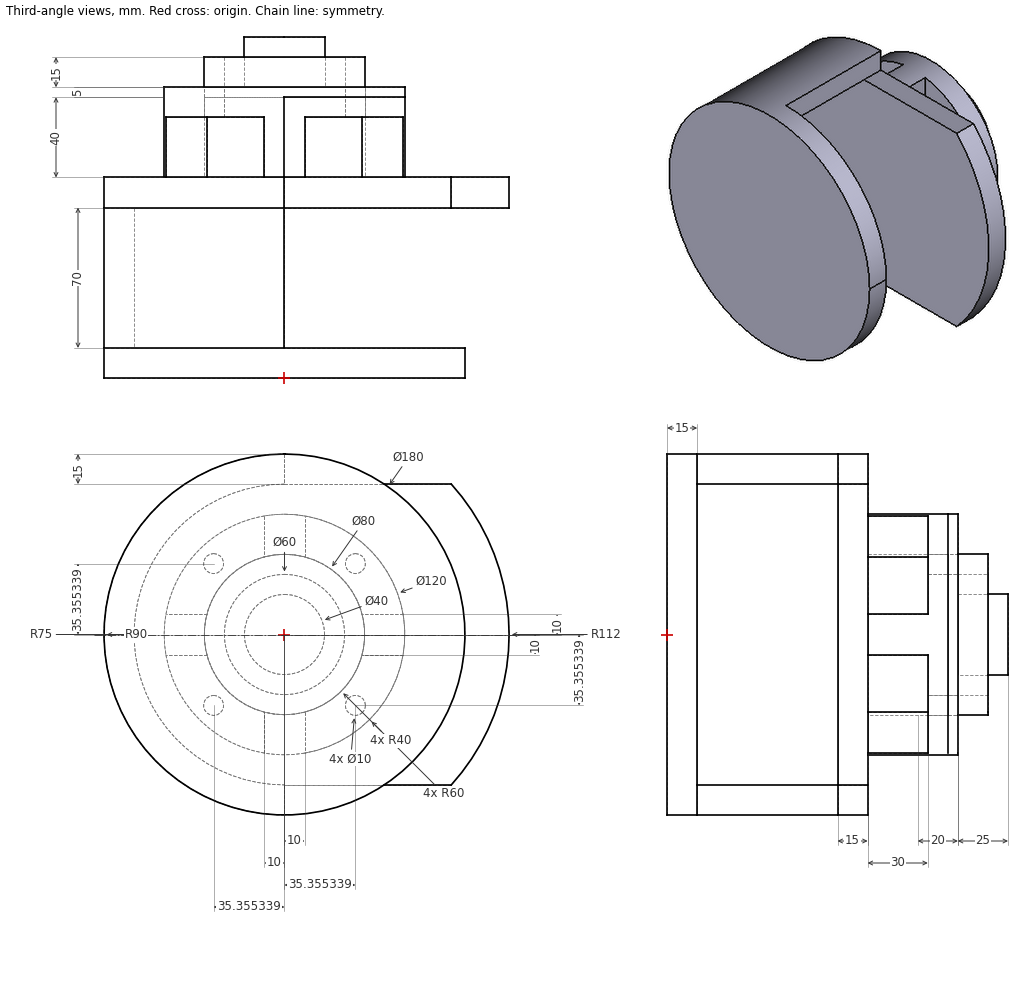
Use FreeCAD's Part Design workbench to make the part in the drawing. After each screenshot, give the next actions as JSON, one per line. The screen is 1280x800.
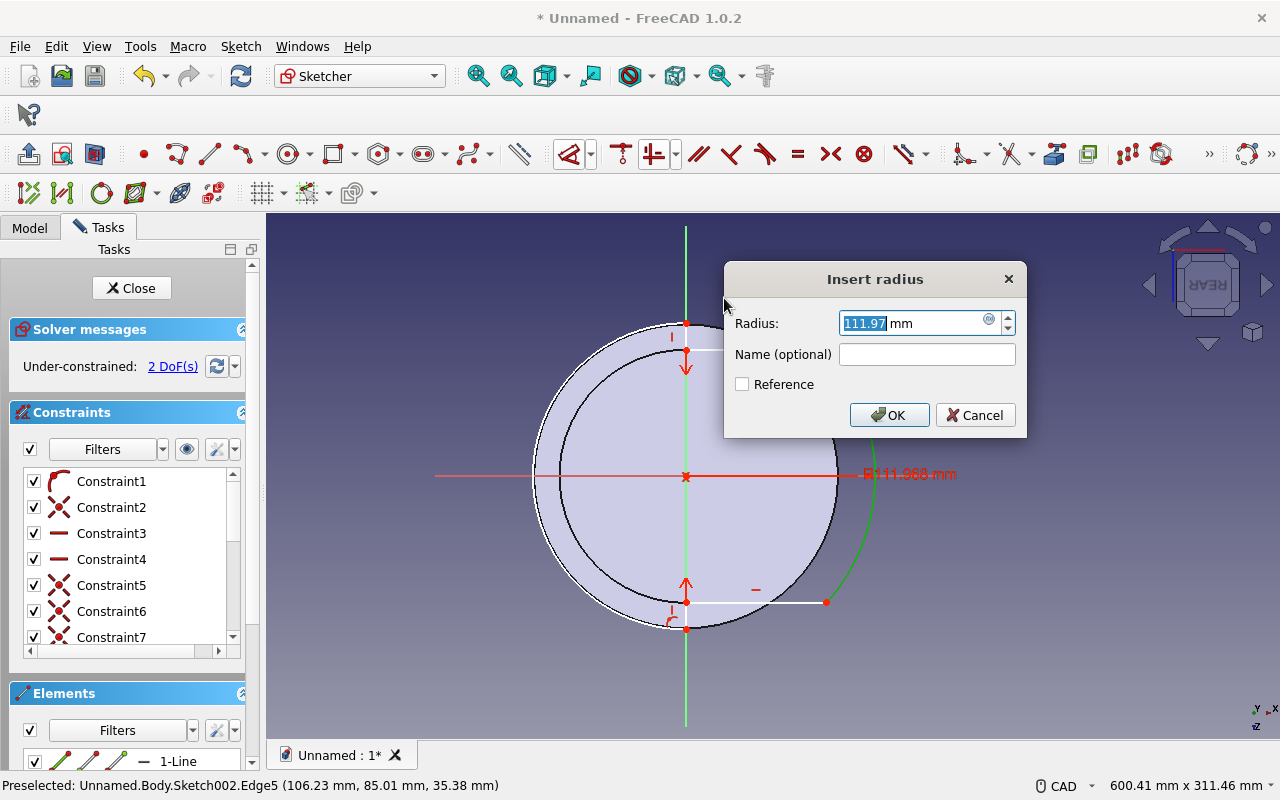
{"action": "type", "text": "112"}
{"action": "key", "text": "Return"}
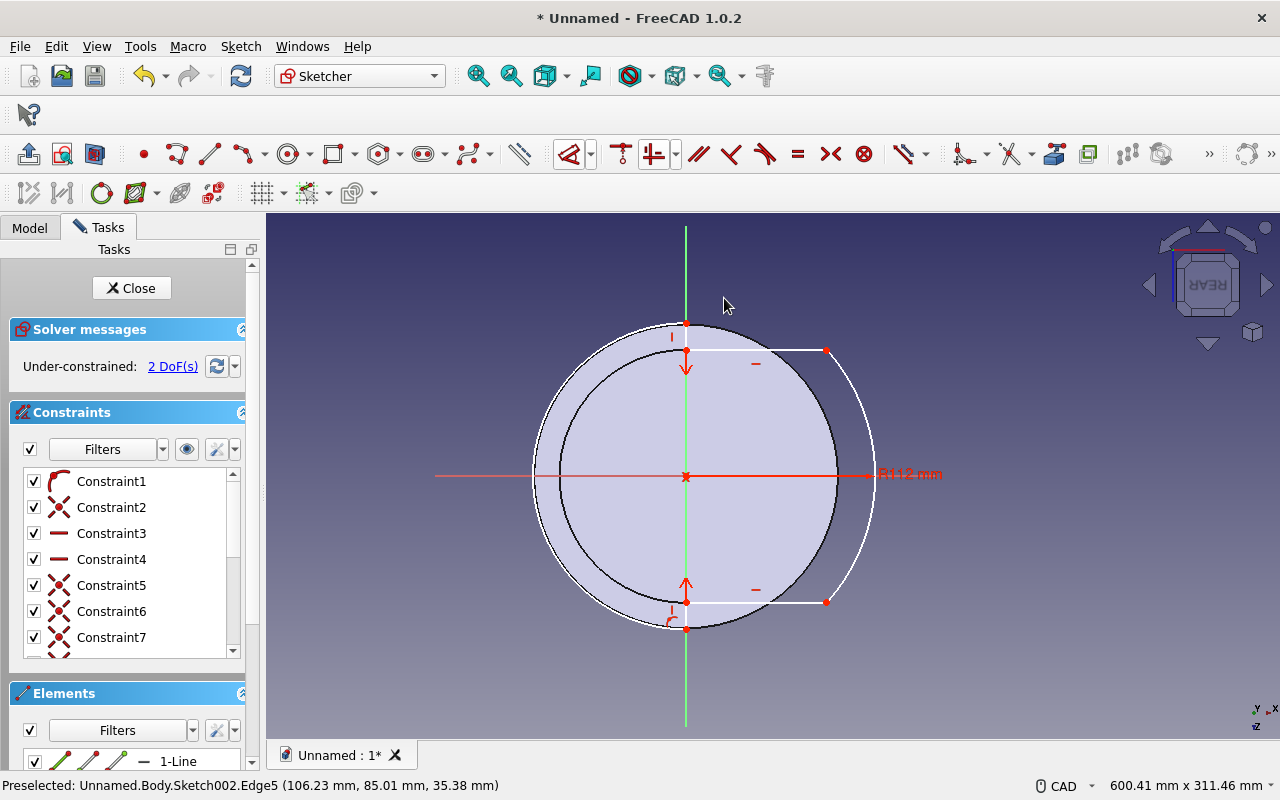
{"action": "left_click", "coordinate": [562, 386]}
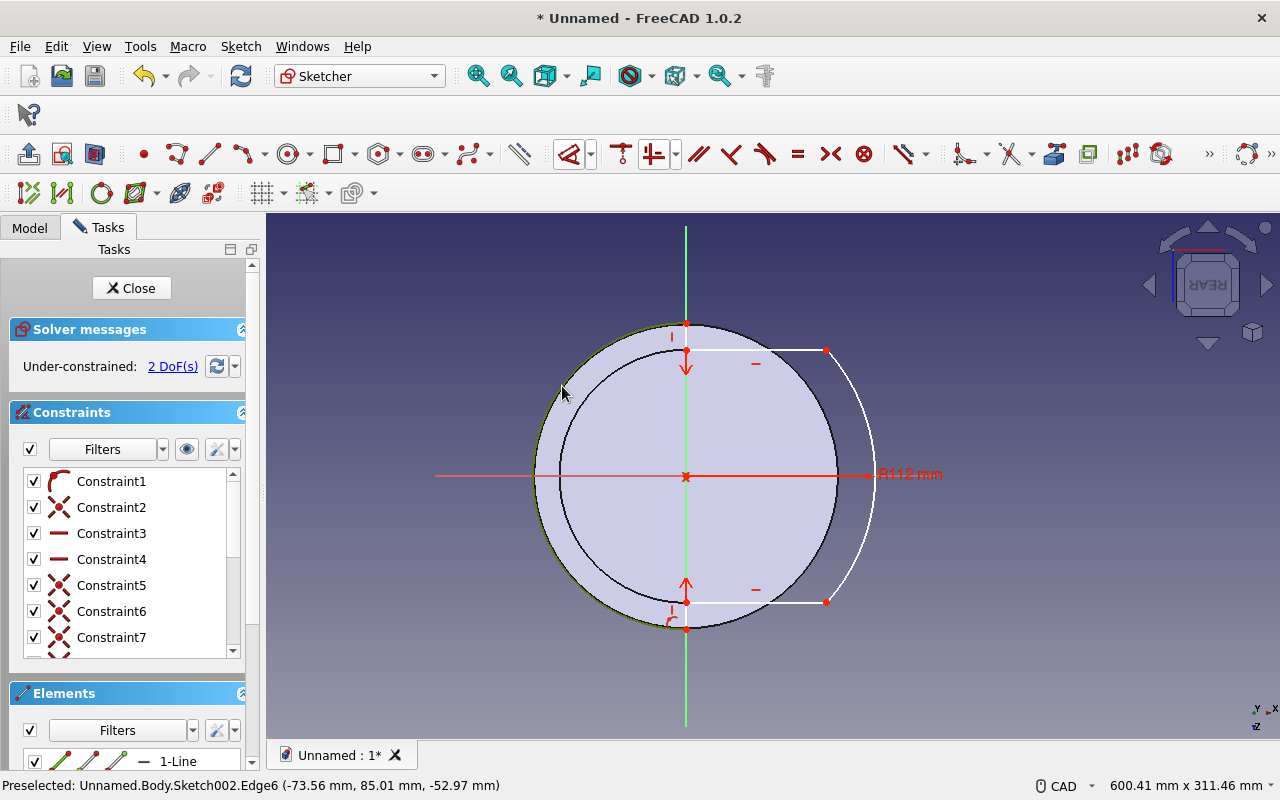
{"action": "key", "text": "k r"}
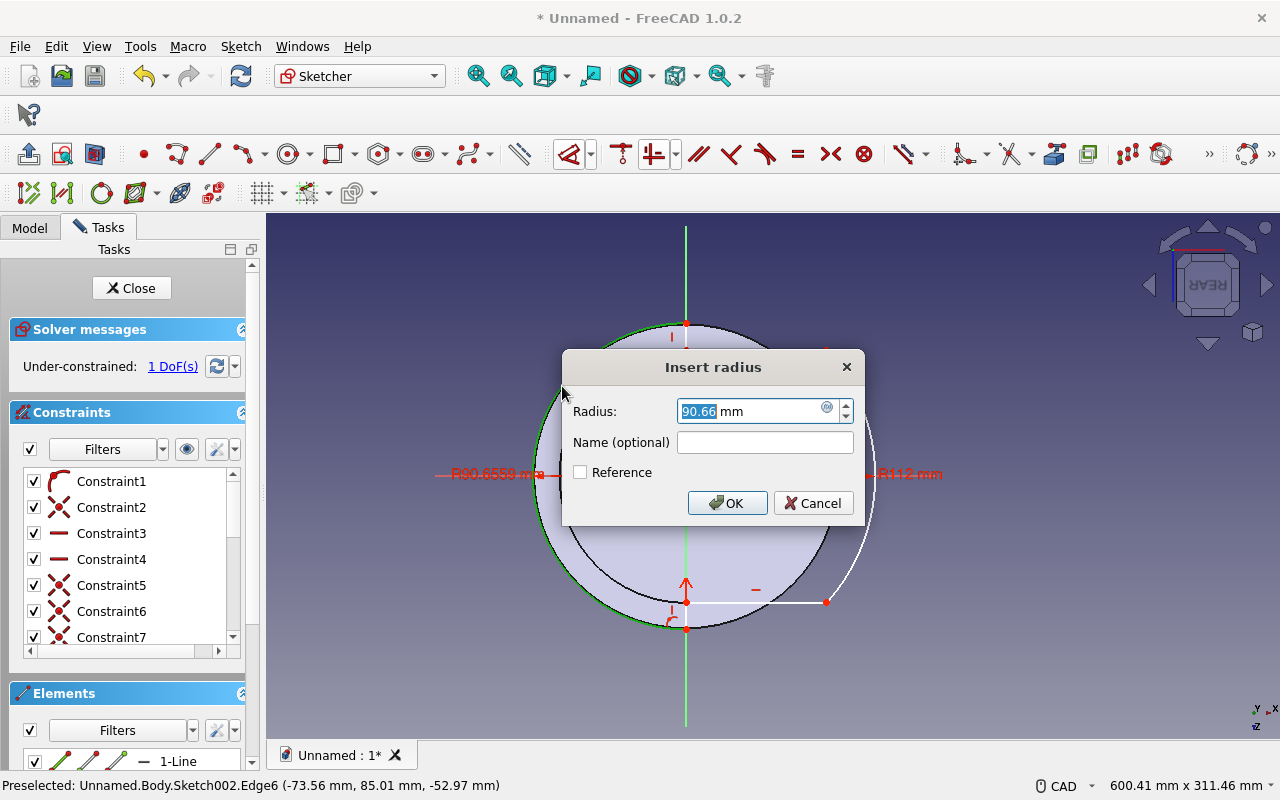
{"action": "type", "text": "90"}
{"action": "key", "text": "Return"}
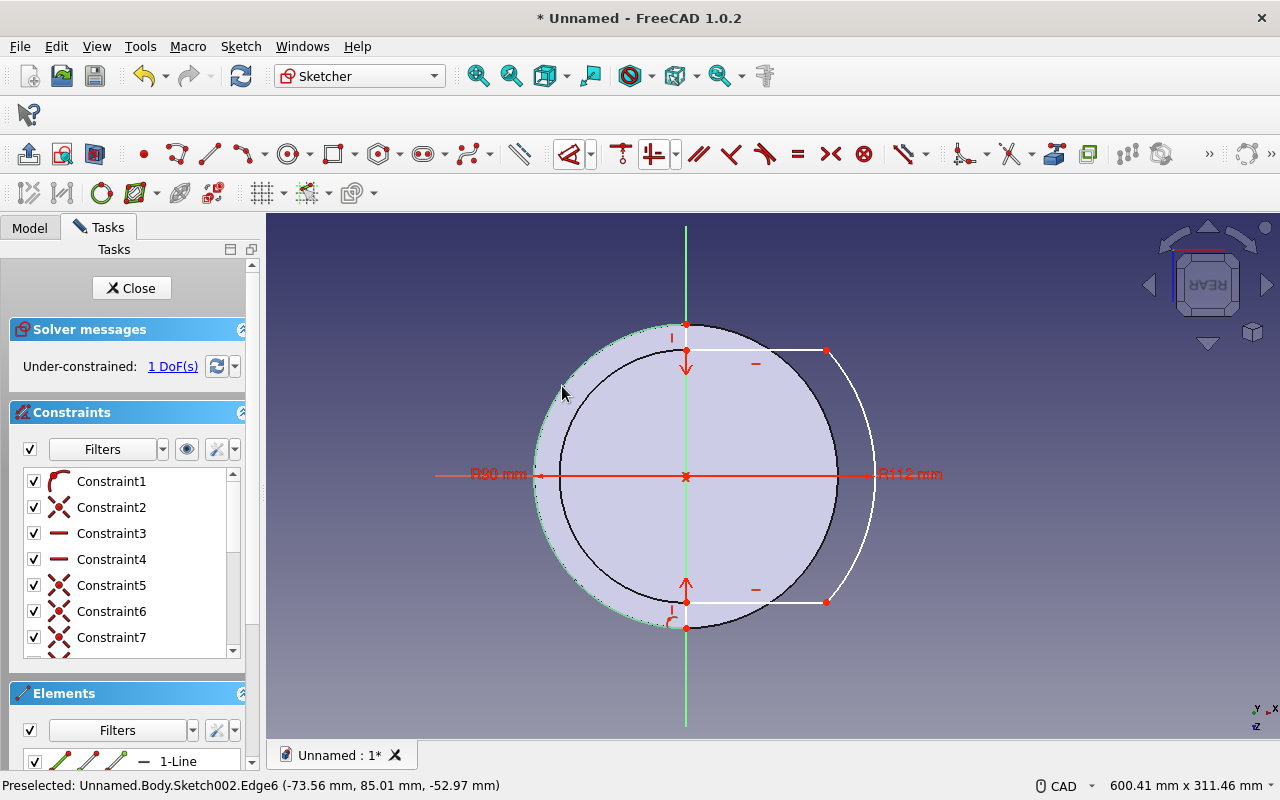
{"action": "scroll", "coordinate": [686, 618], "scroll_direction": "up", "scroll_amount": 3}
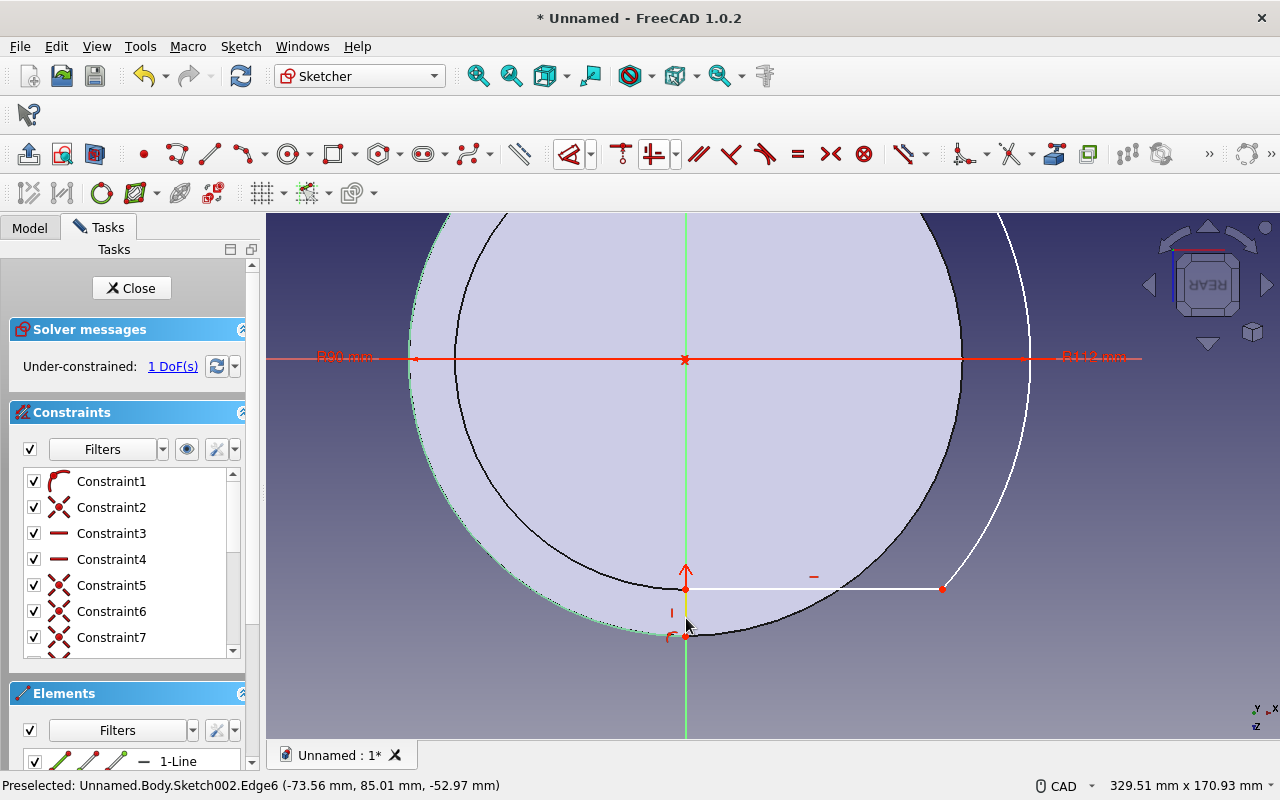
{"action": "left_click", "coordinate": [686, 617]}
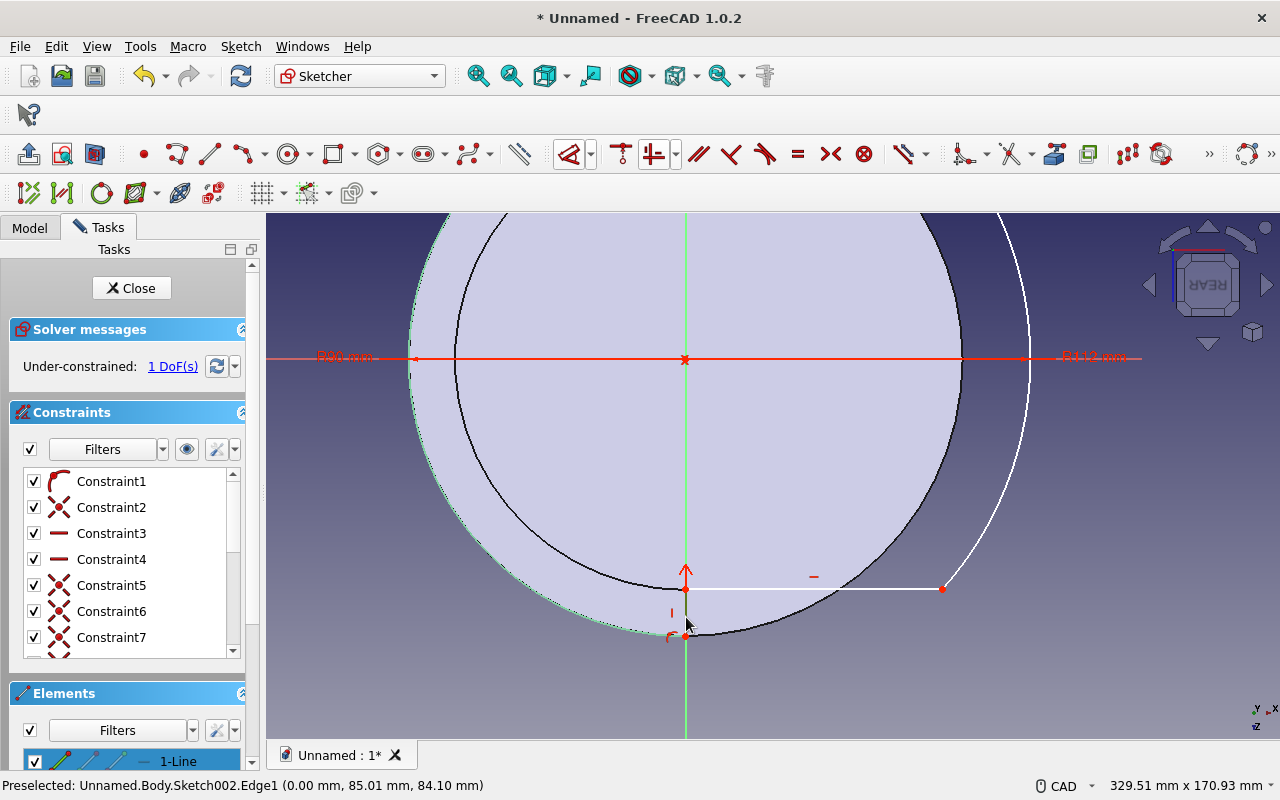
{"action": "key", "text": "i"}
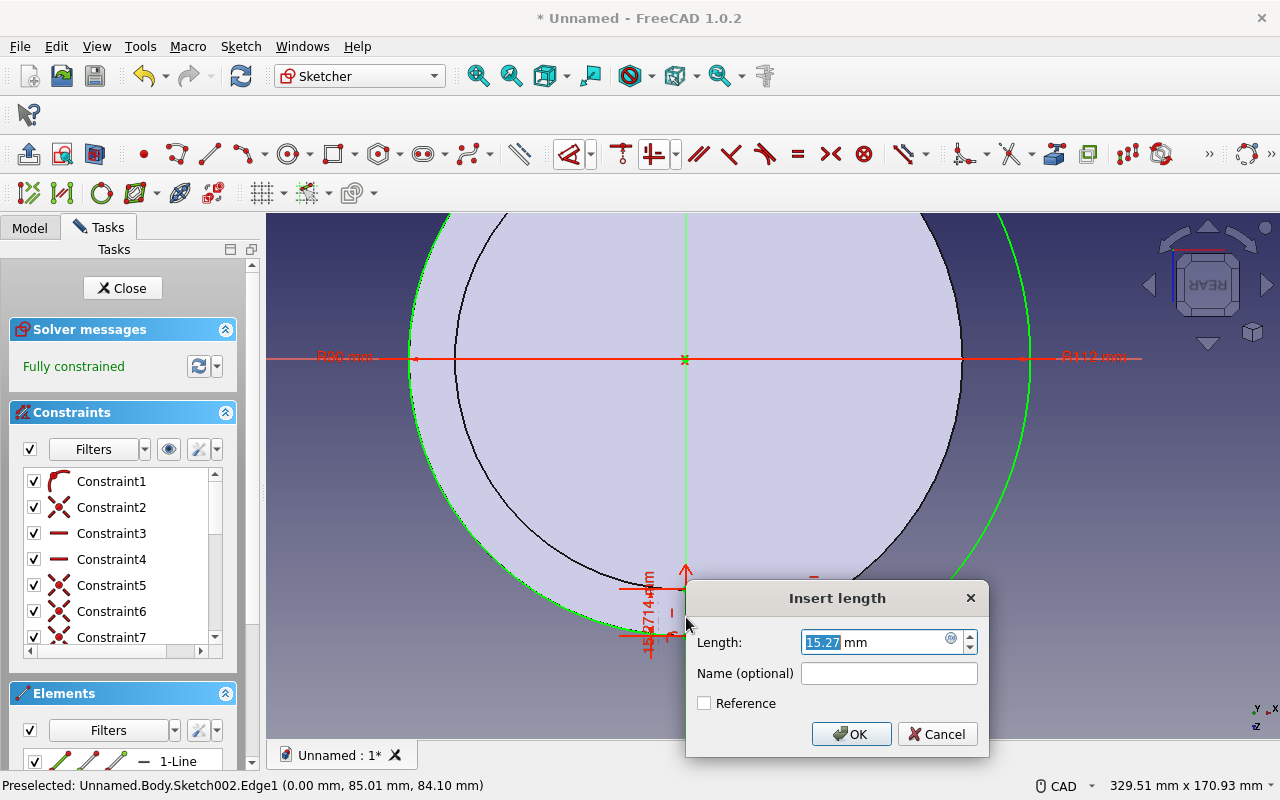
{"action": "type", "text": "15"}
{"action": "key", "text": "Return"}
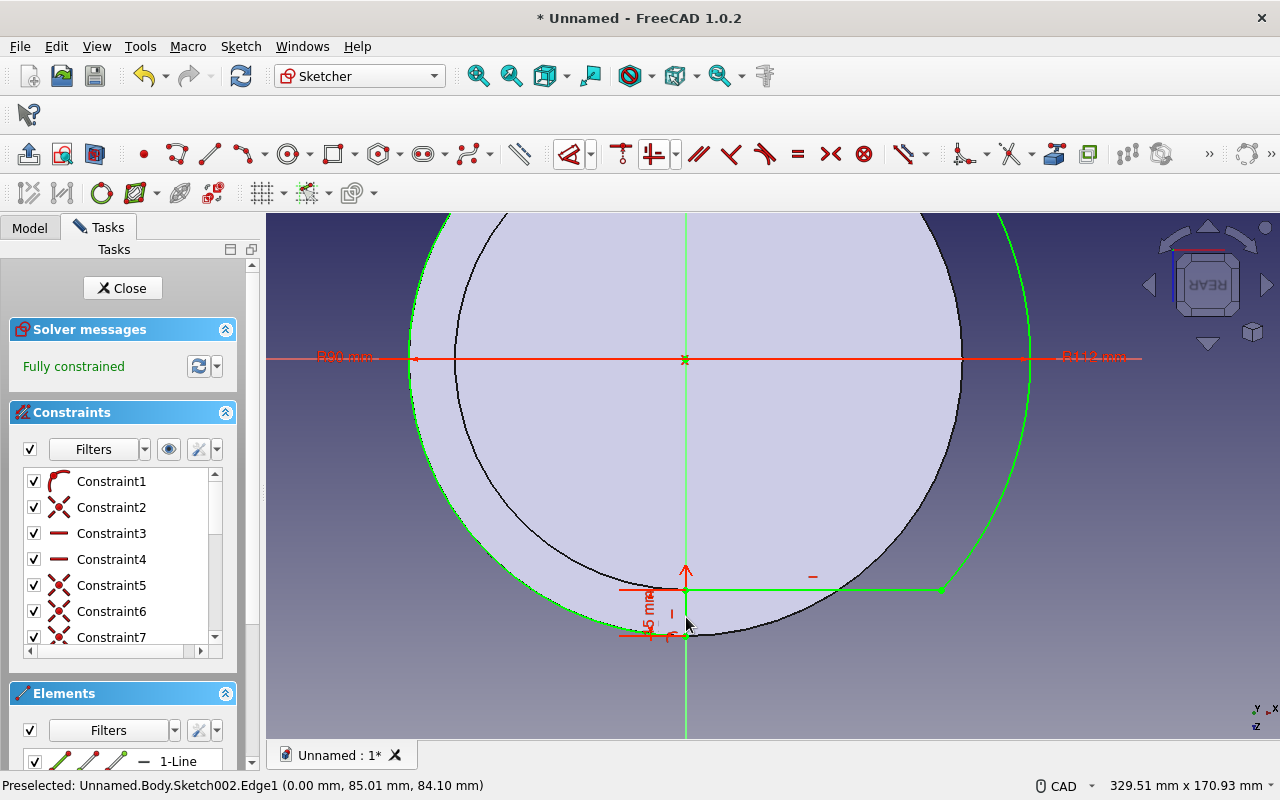
{"action": "left_click", "coordinate": [123, 288]}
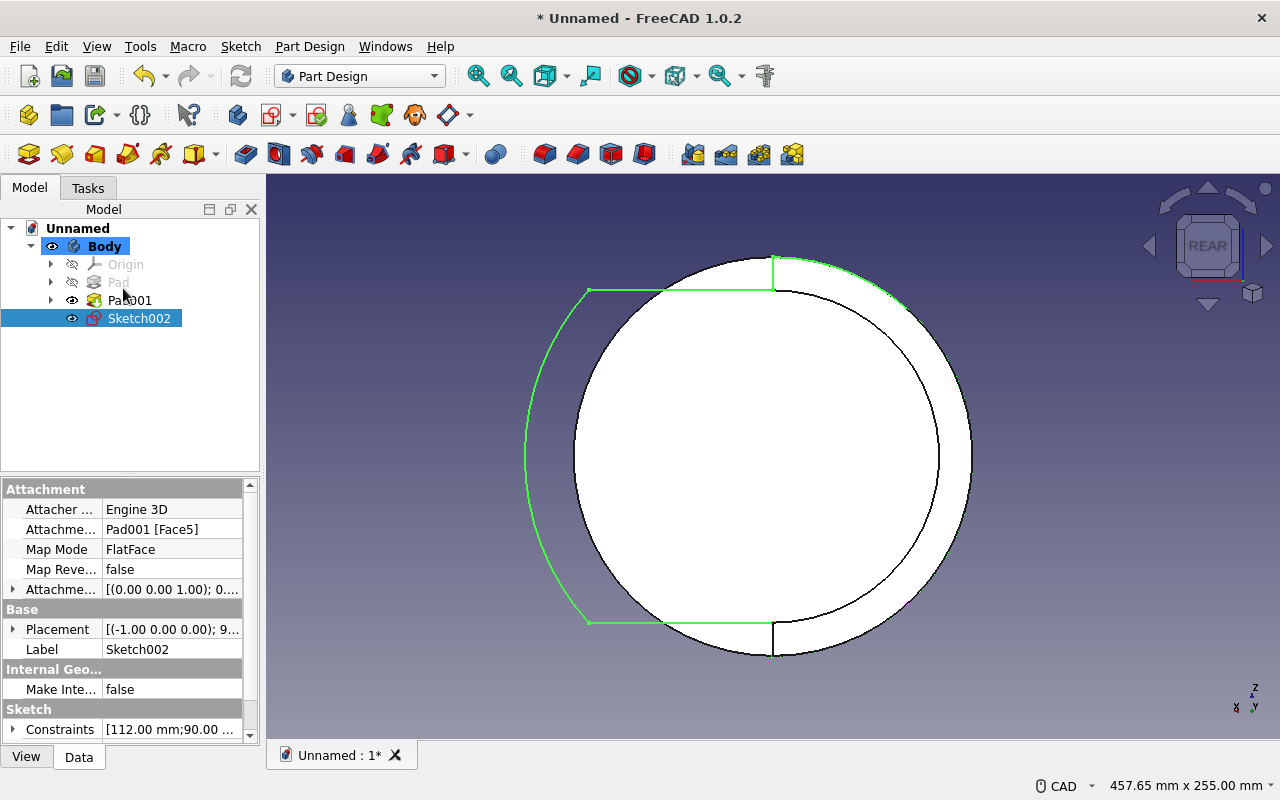
{"action": "left_click", "coordinate": [29, 154]}